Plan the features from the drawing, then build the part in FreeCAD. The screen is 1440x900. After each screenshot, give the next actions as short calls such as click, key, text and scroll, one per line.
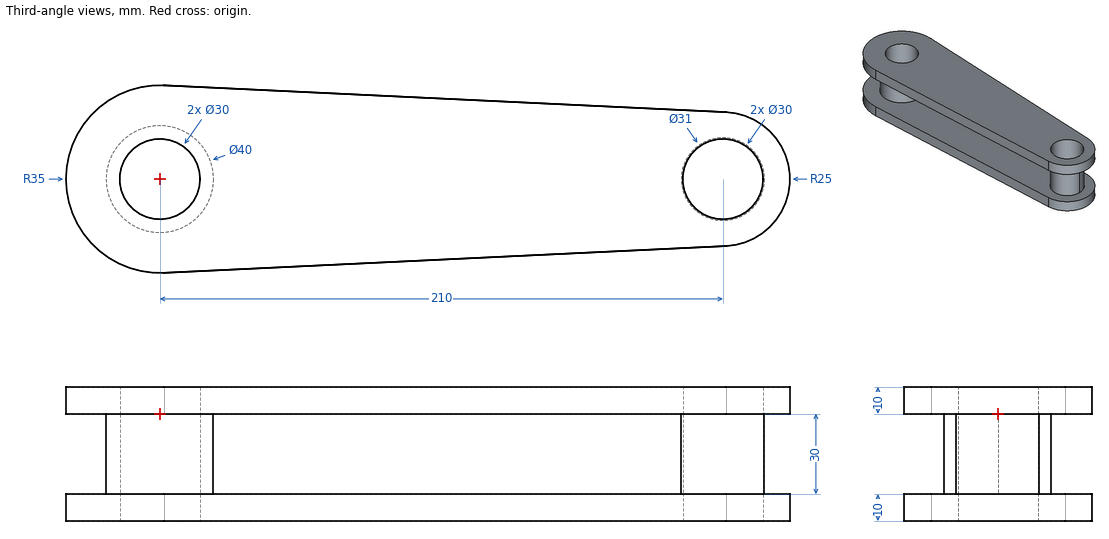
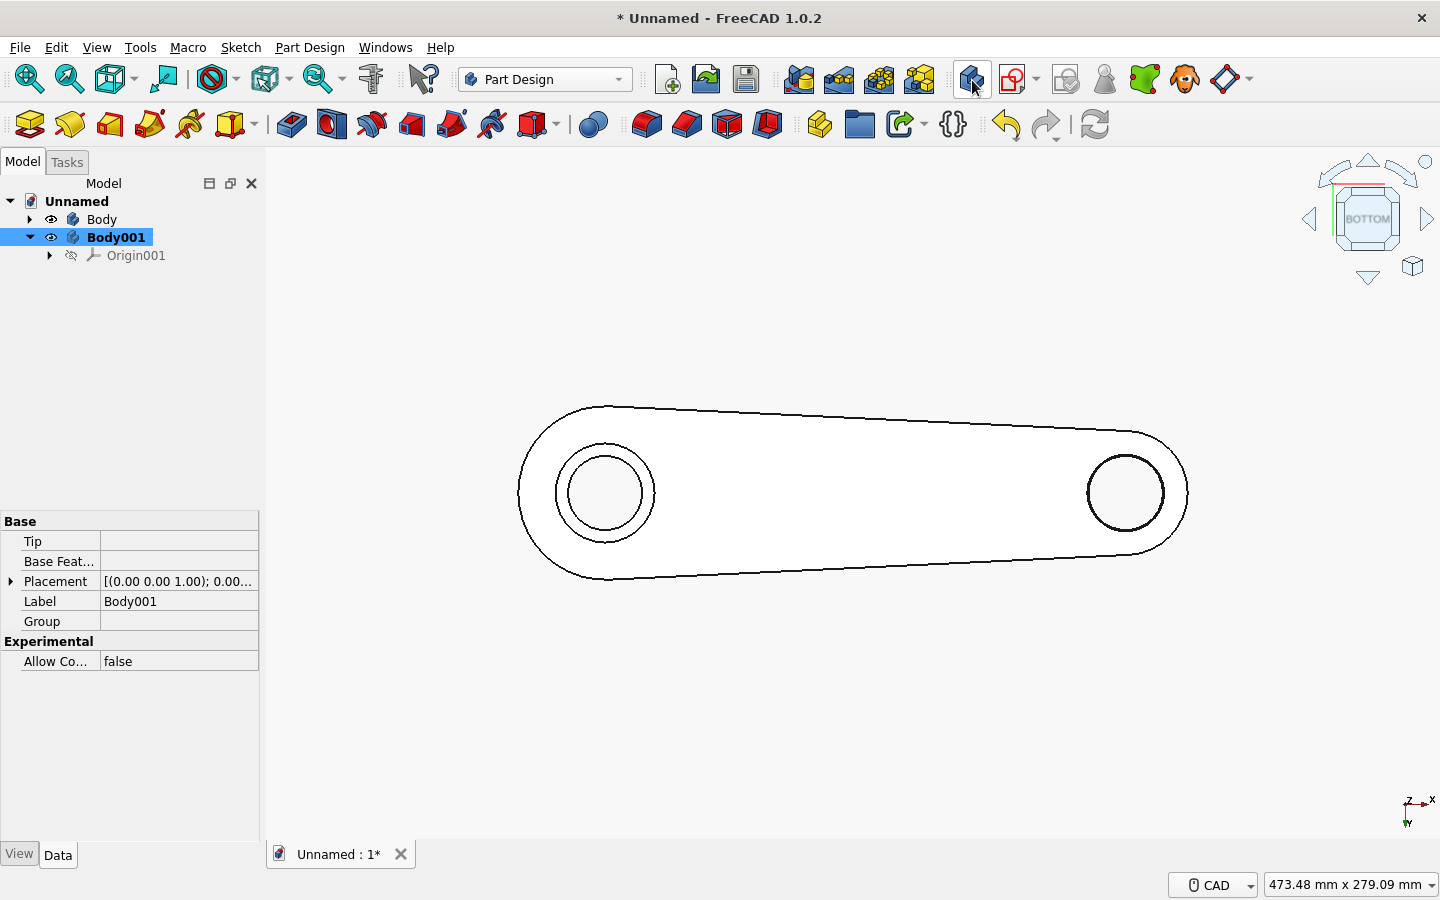
click(50, 255)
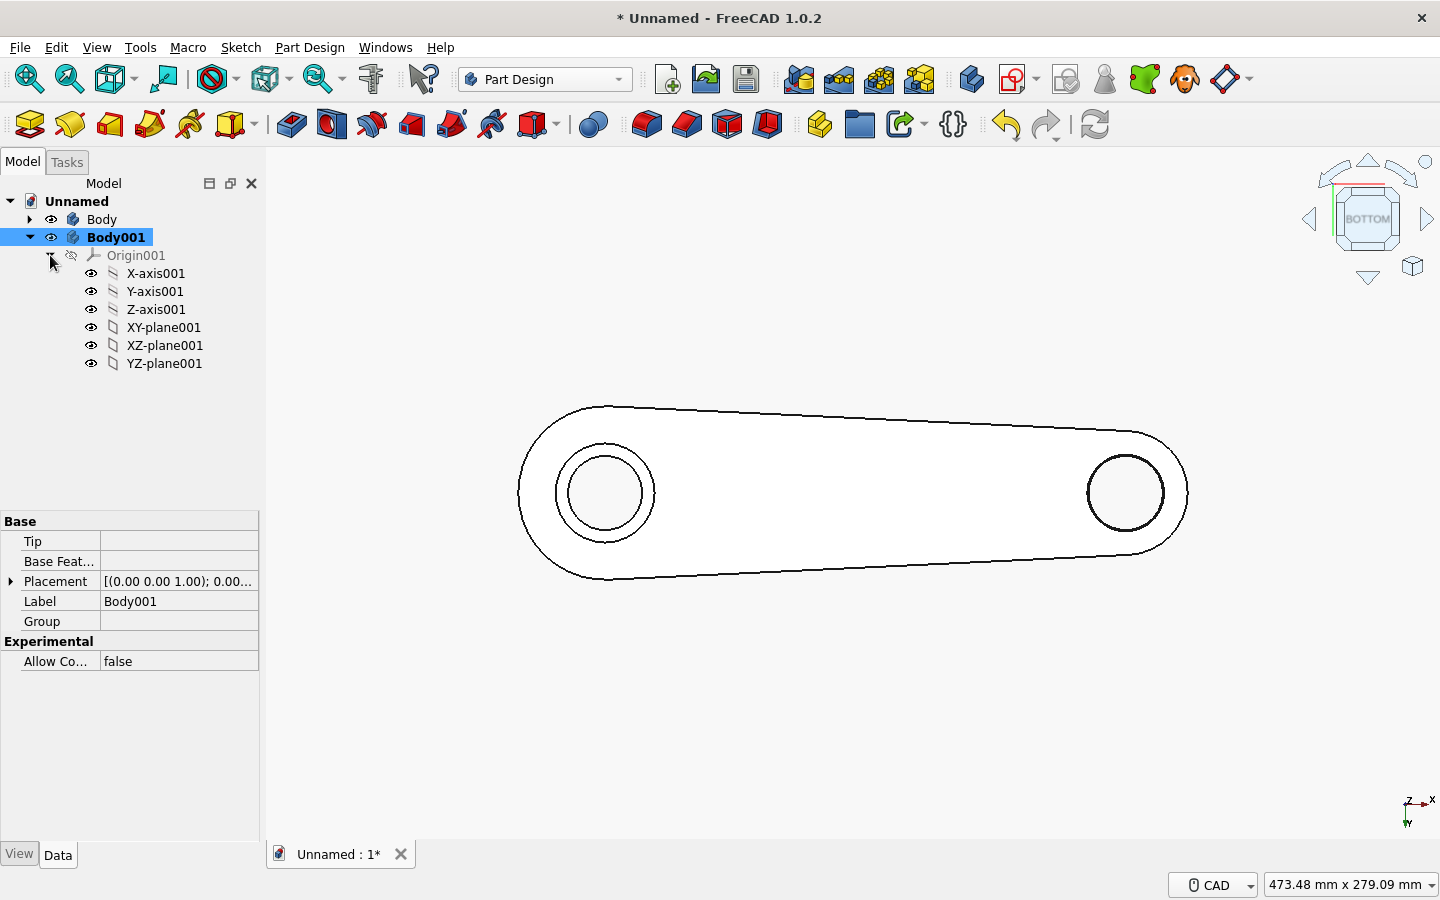
click(136, 327)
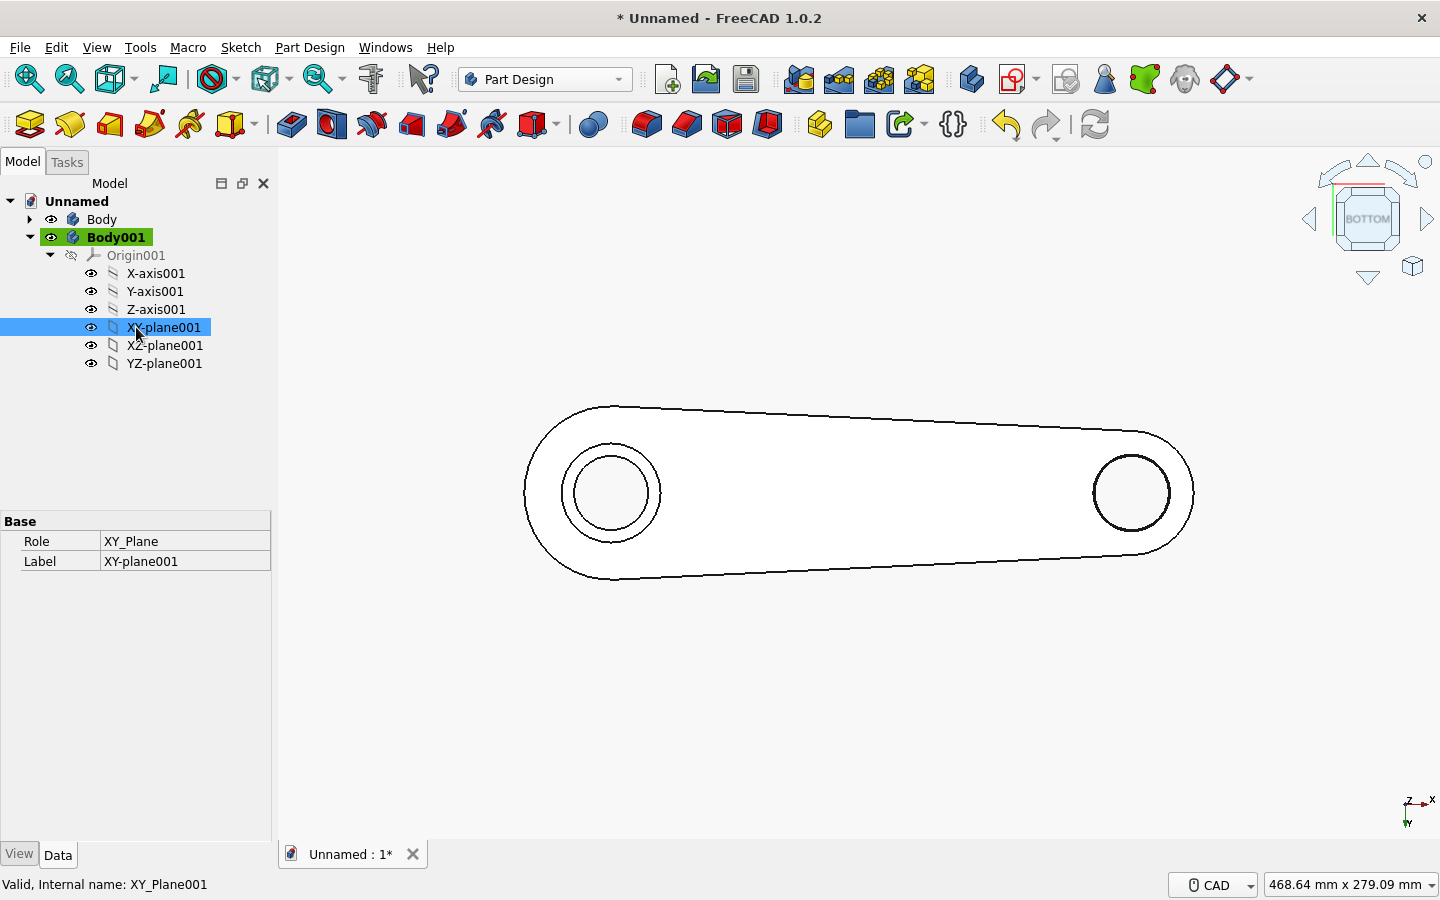
click(1226, 80)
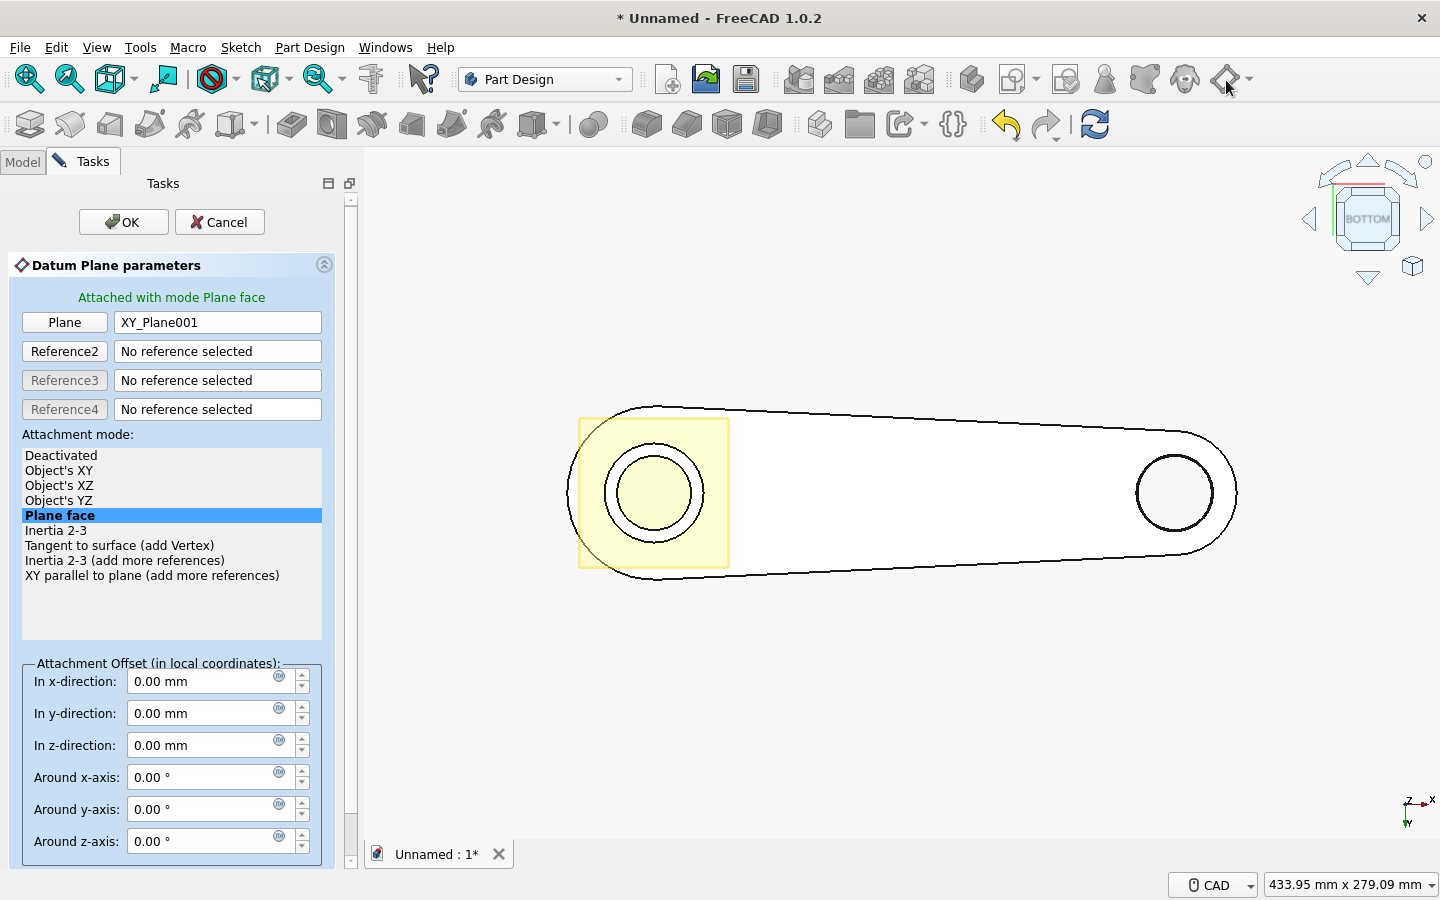
triple_click(210, 745)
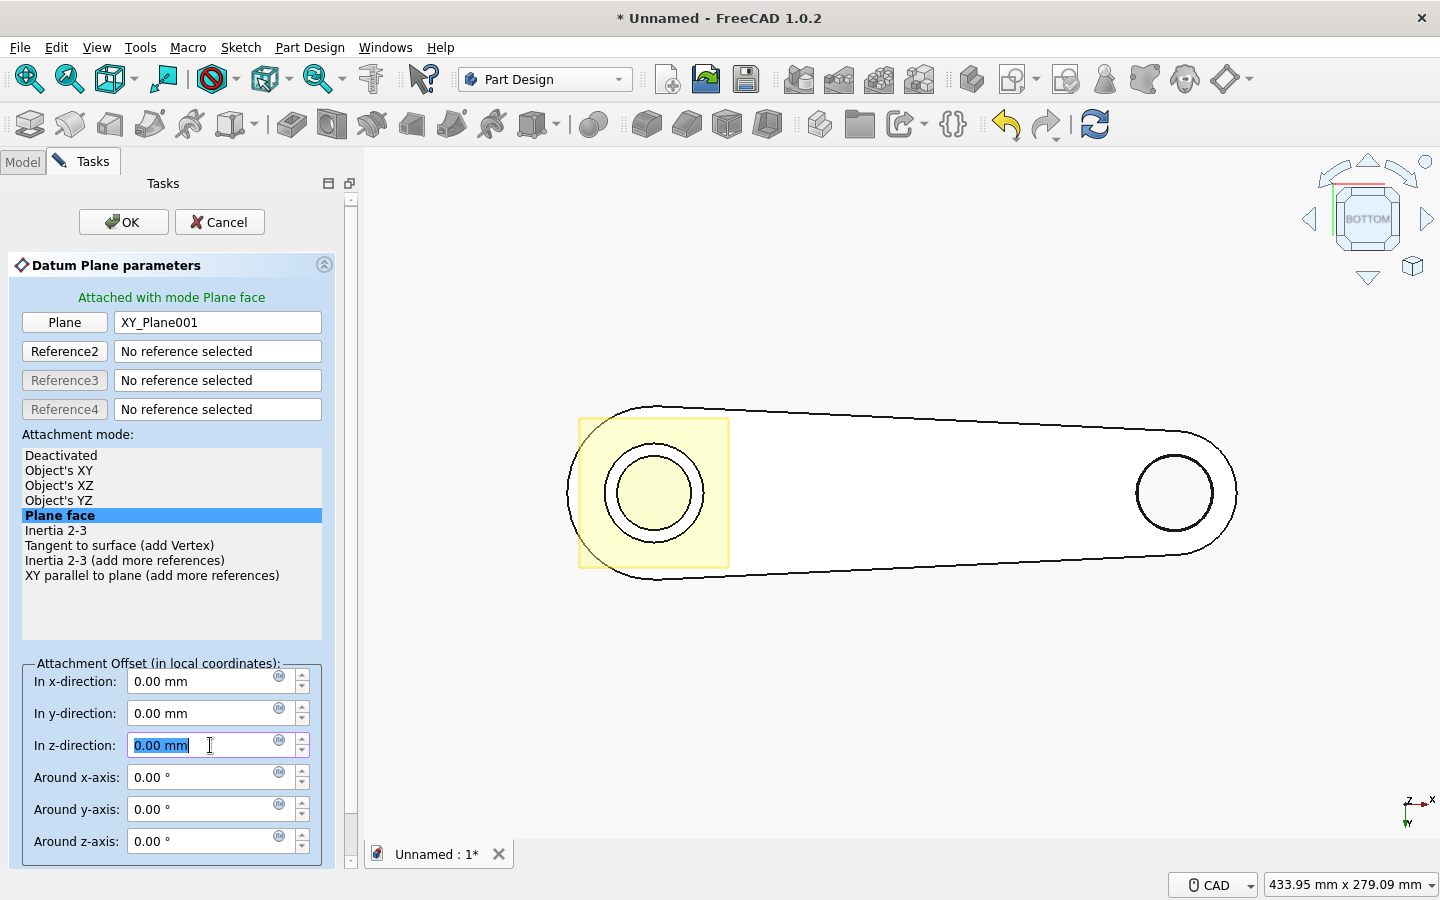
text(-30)
key(Tab)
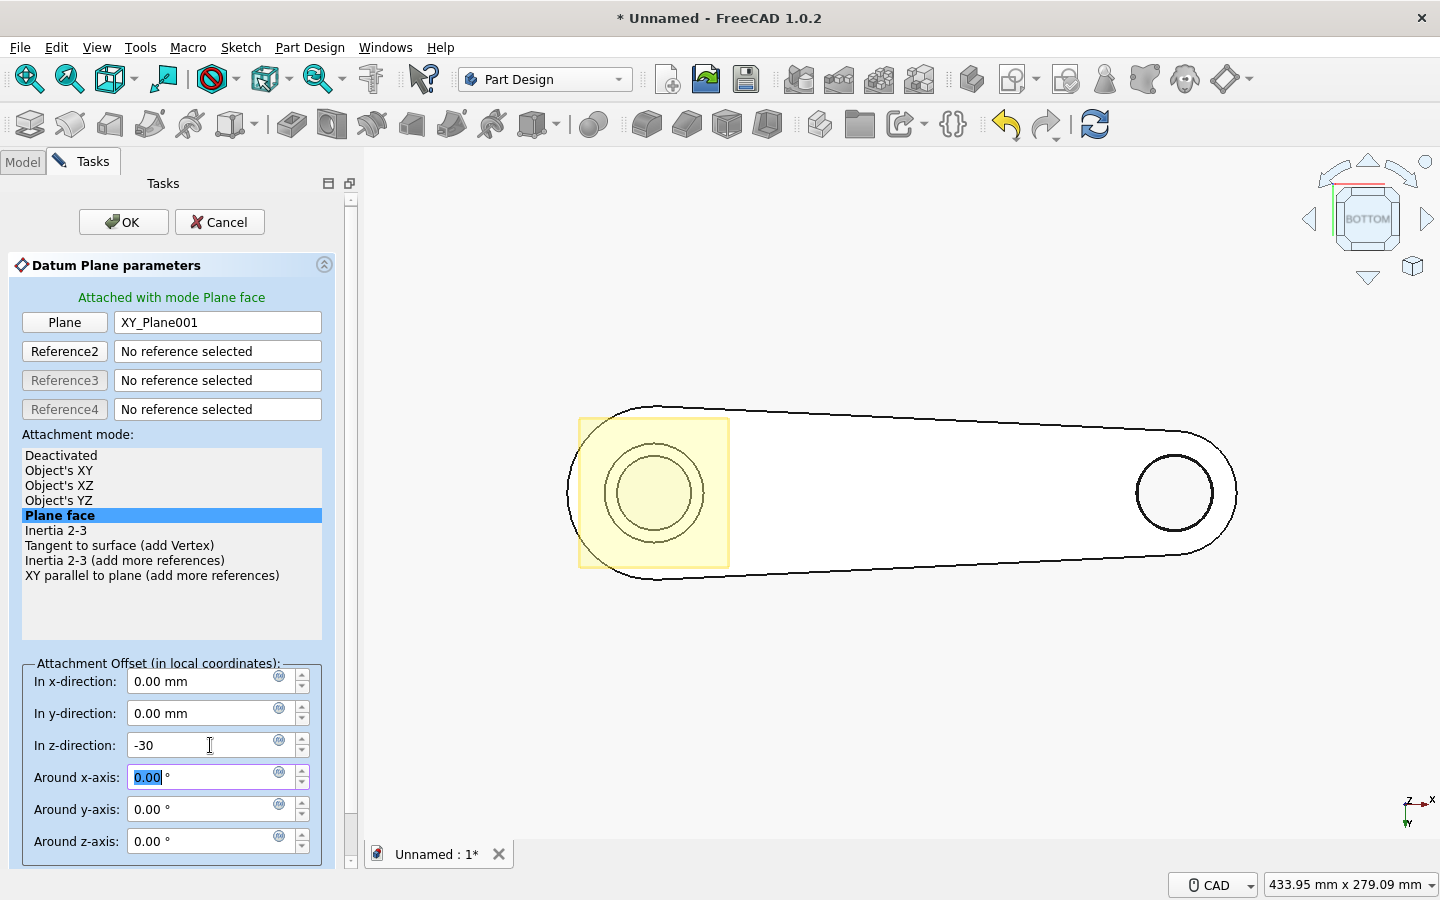
click(124, 222)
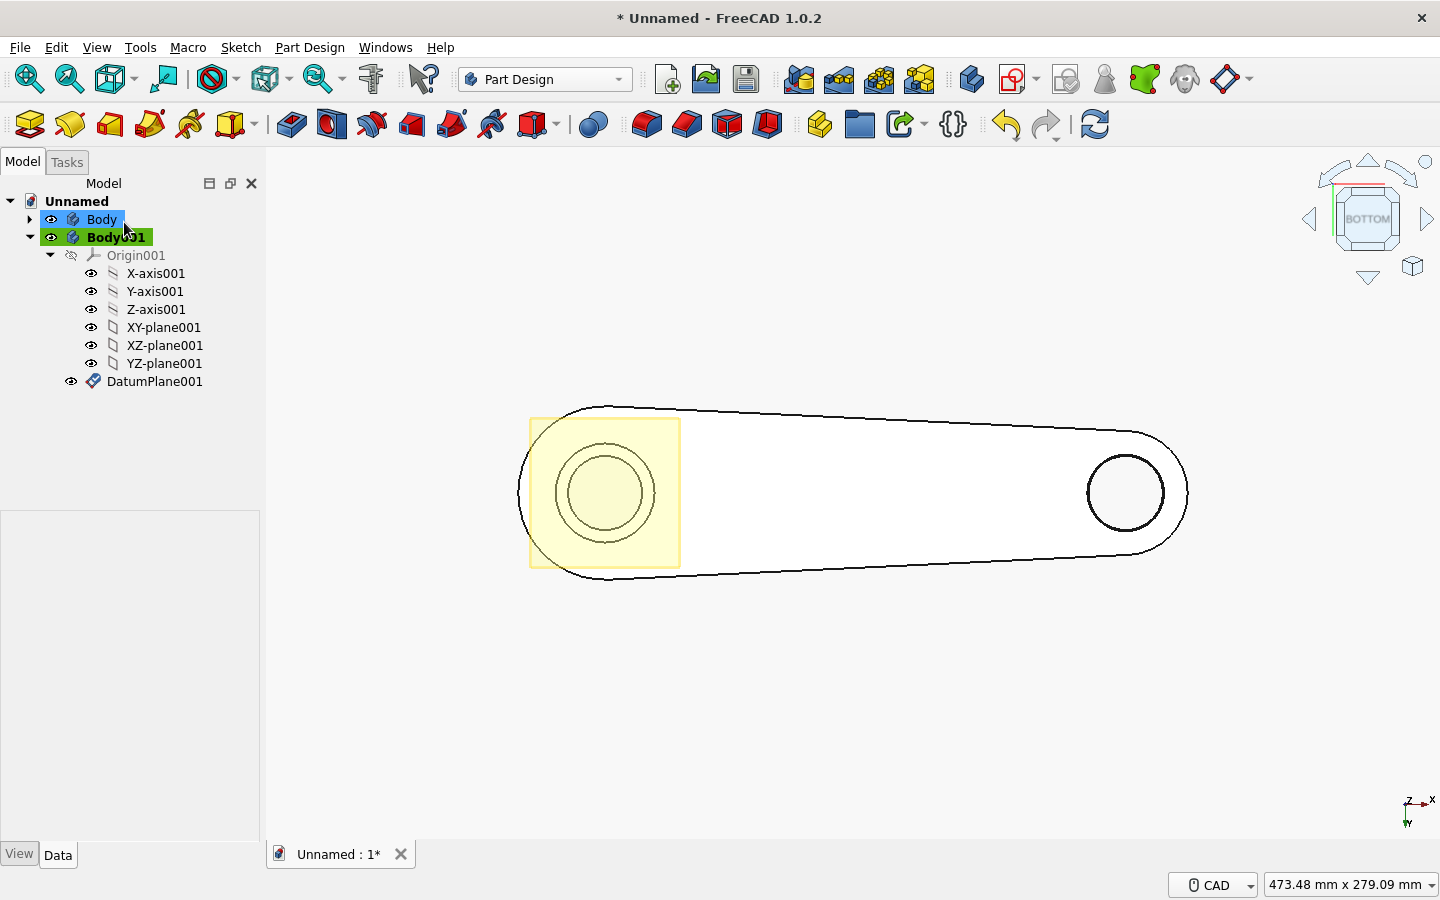
click(116, 381)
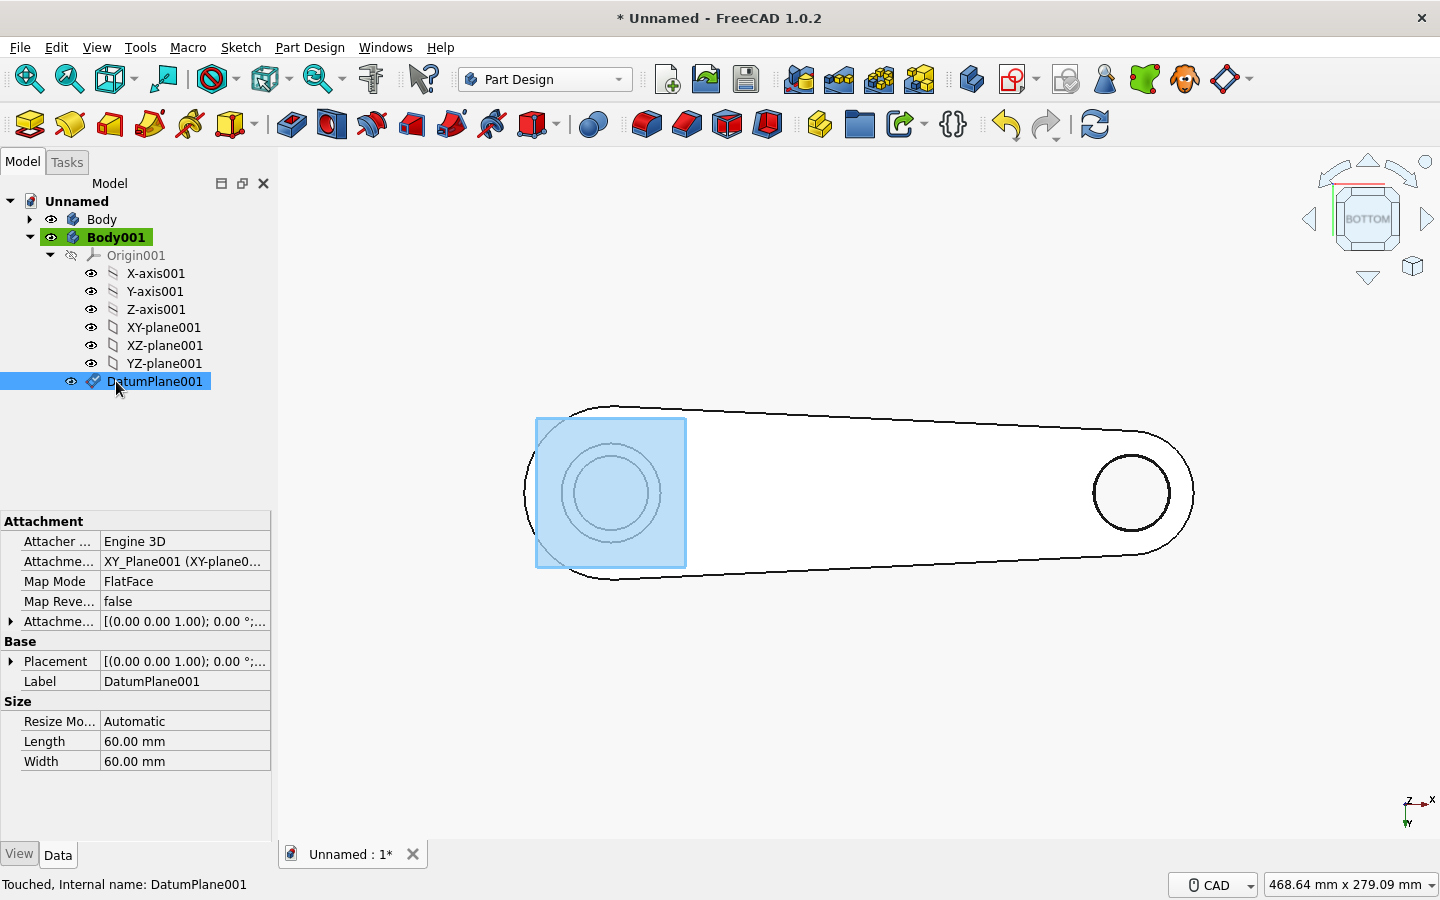
click(1012, 80)